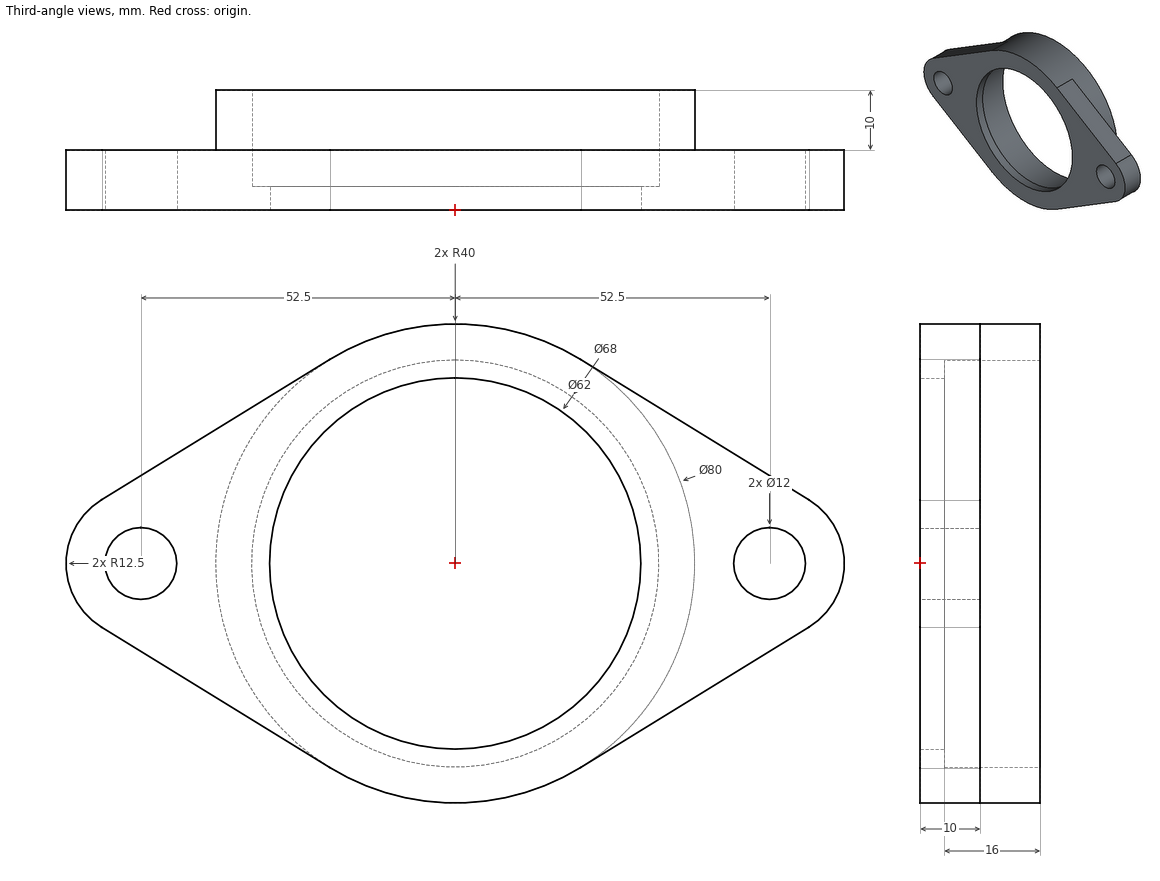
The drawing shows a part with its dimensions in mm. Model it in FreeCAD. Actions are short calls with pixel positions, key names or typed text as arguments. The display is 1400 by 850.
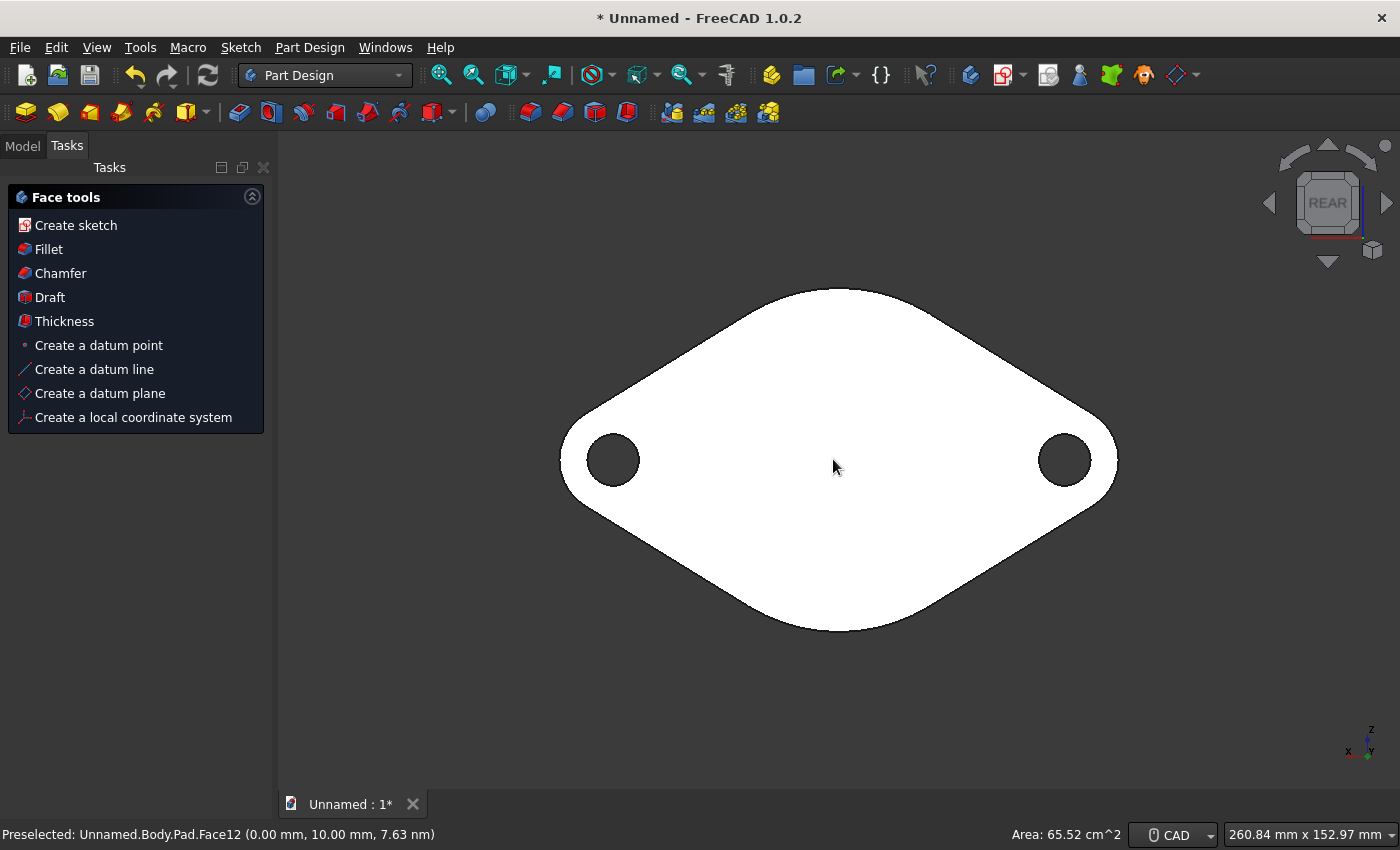
click(1004, 76)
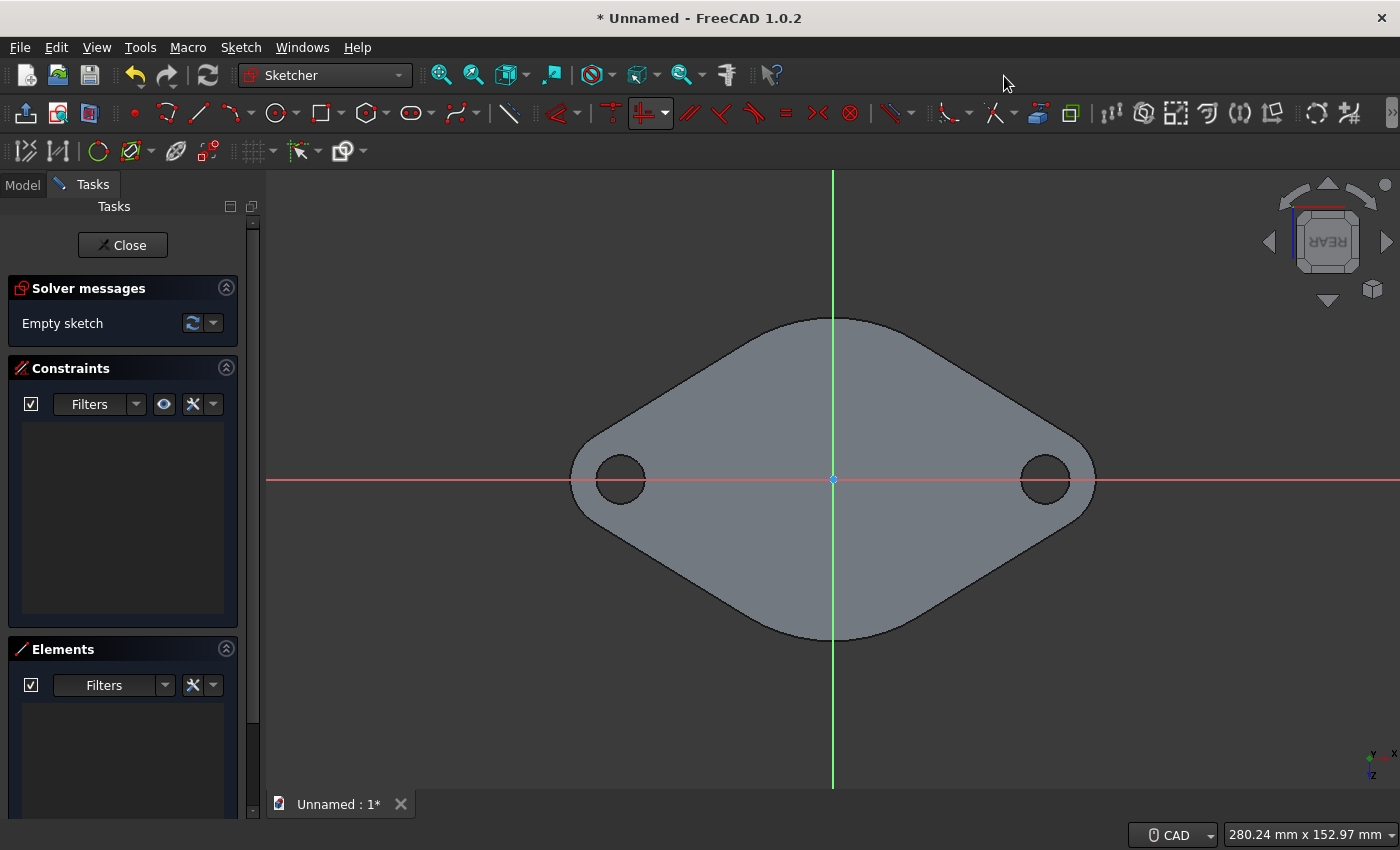
click(276, 114)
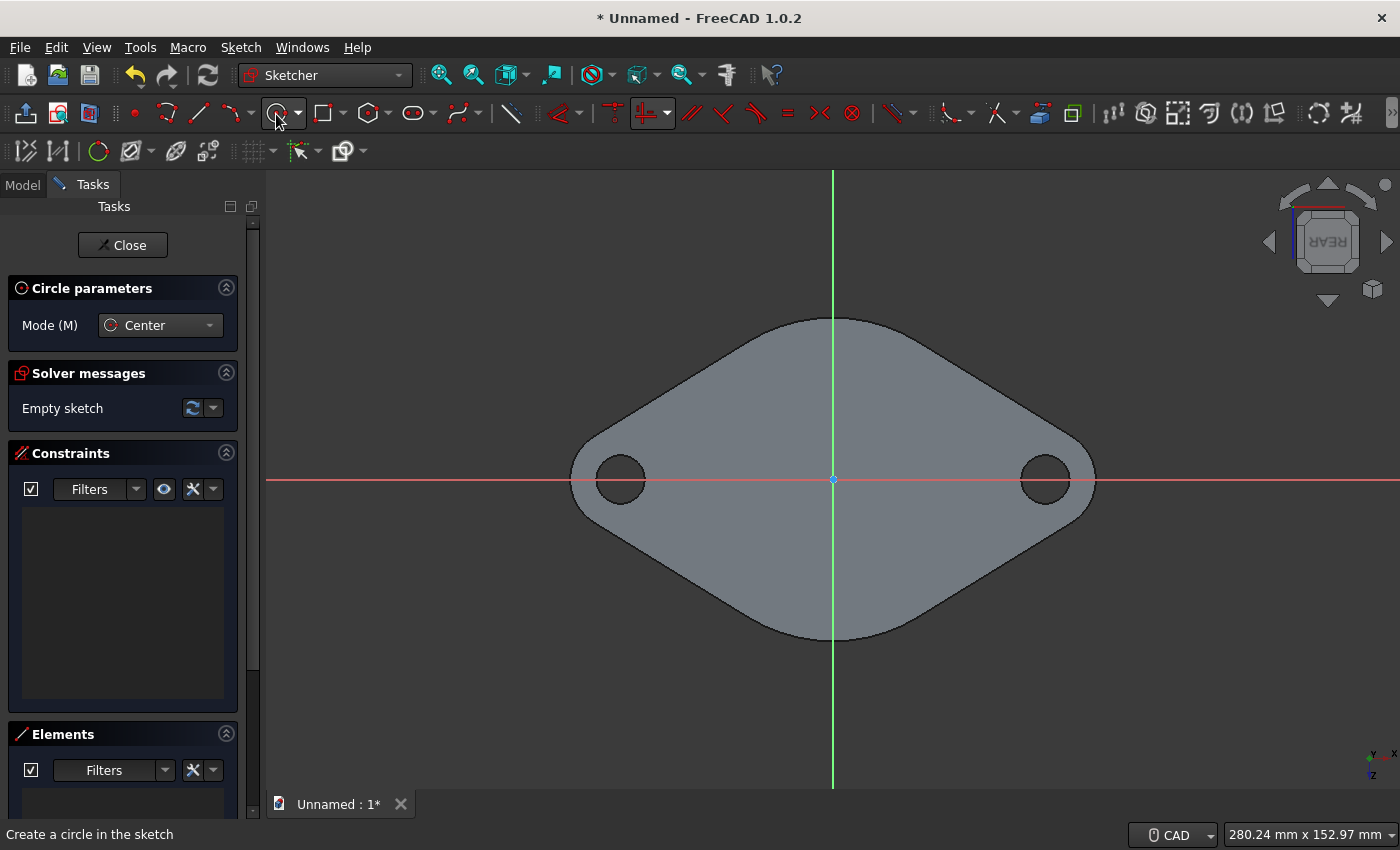
click(833, 479)
move(947, 365)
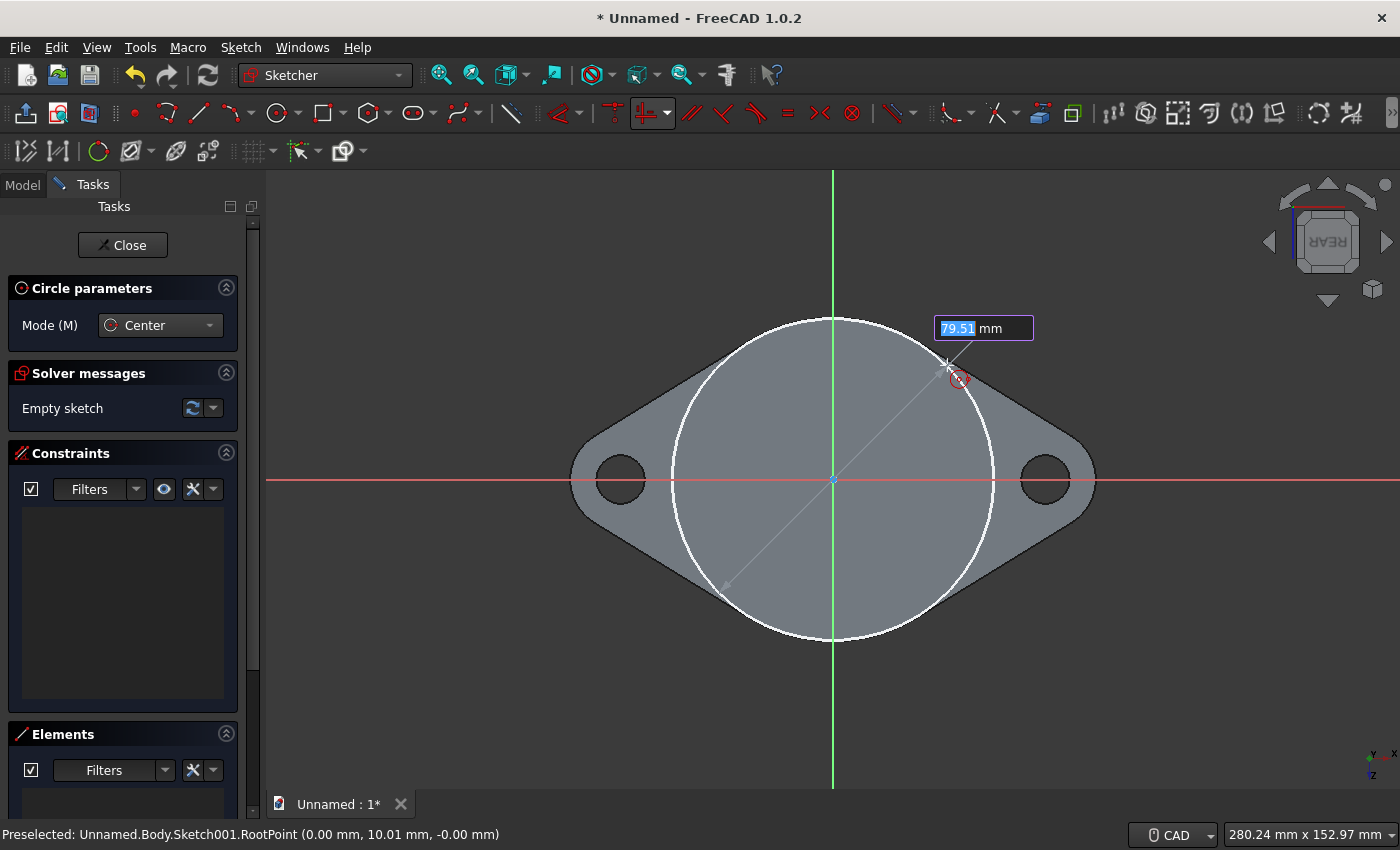
text(80)
key(Return)
key(Escape)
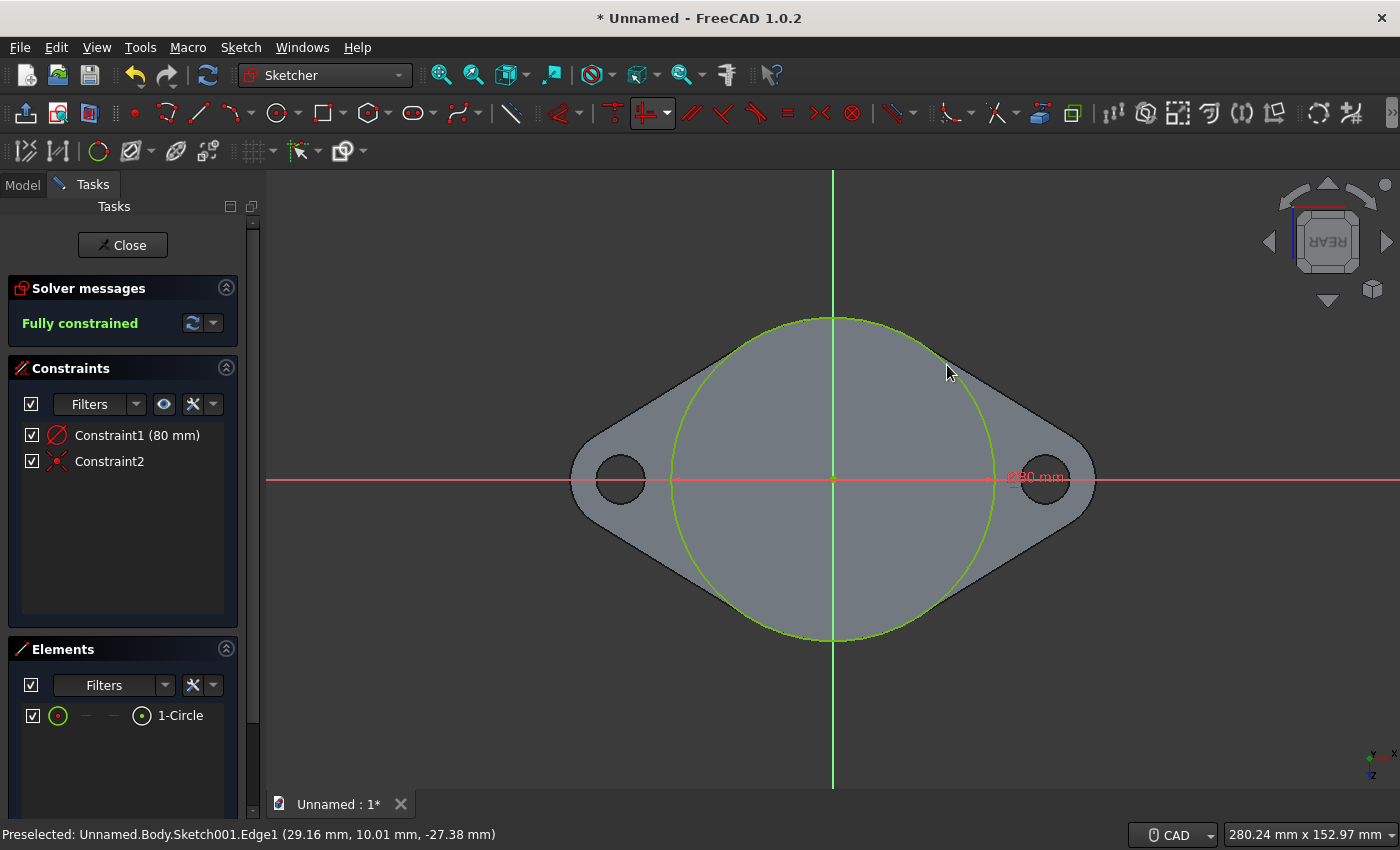
click(123, 245)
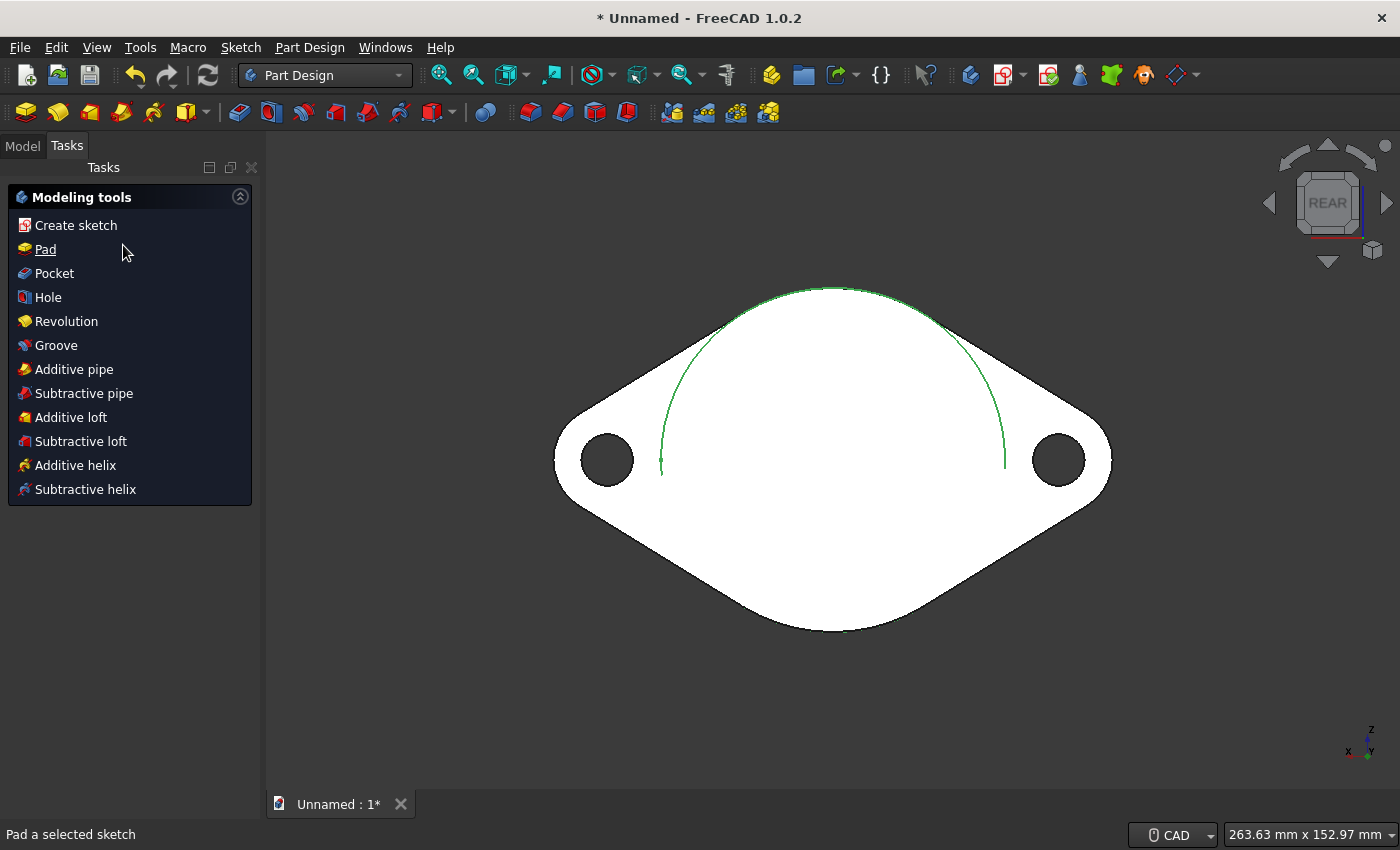
click(26, 112)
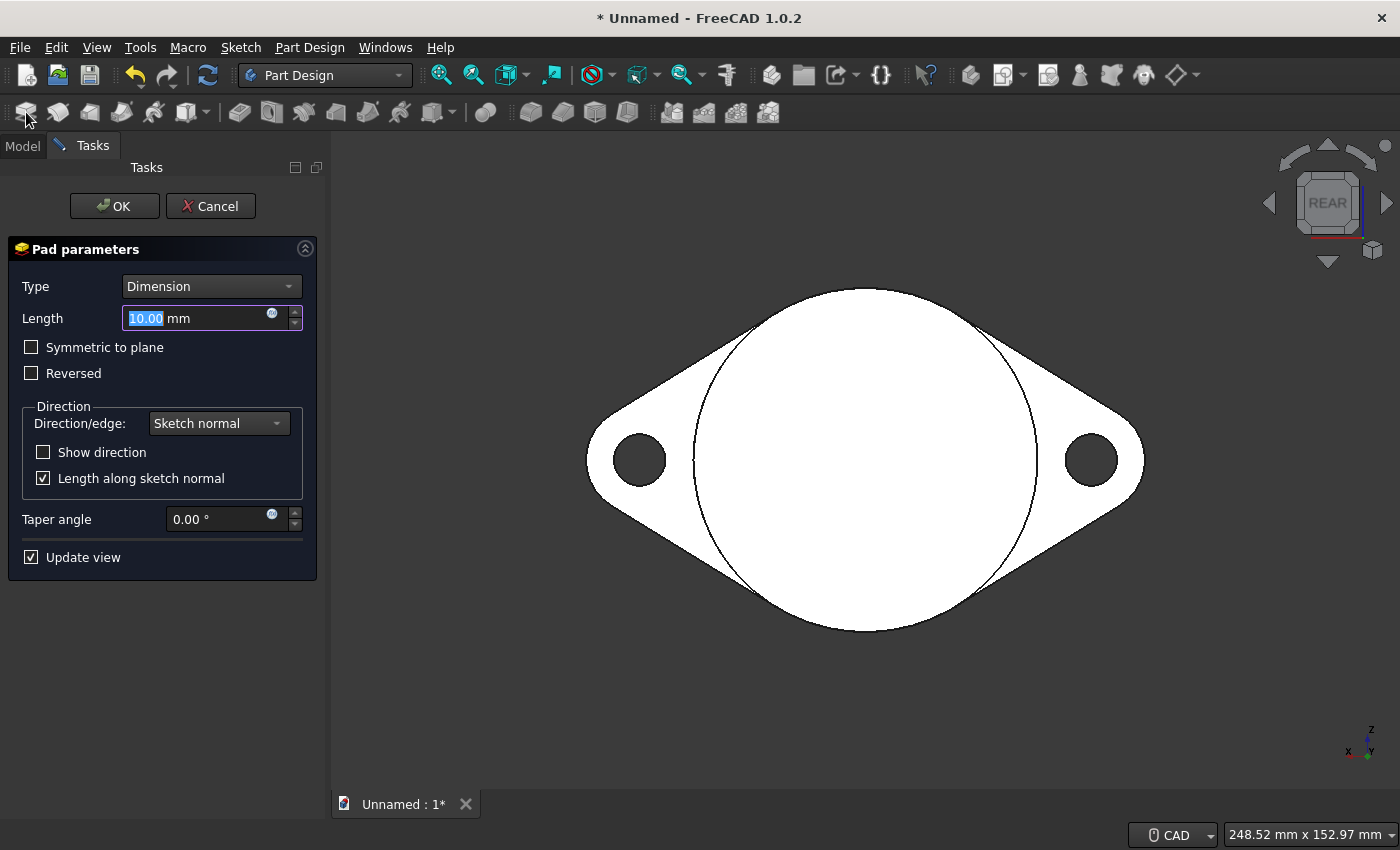
text(10)
key(Tab)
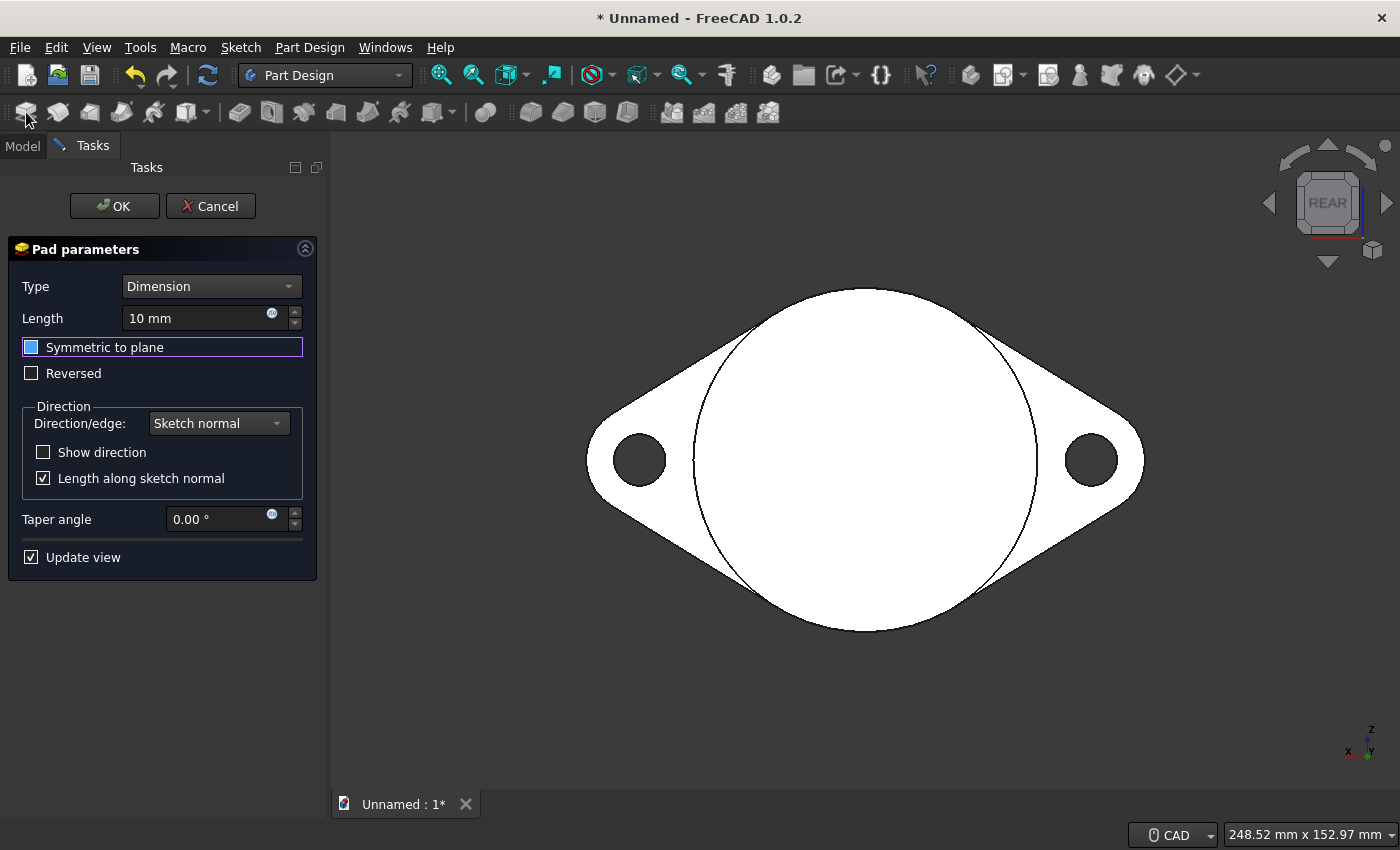
click(115, 206)